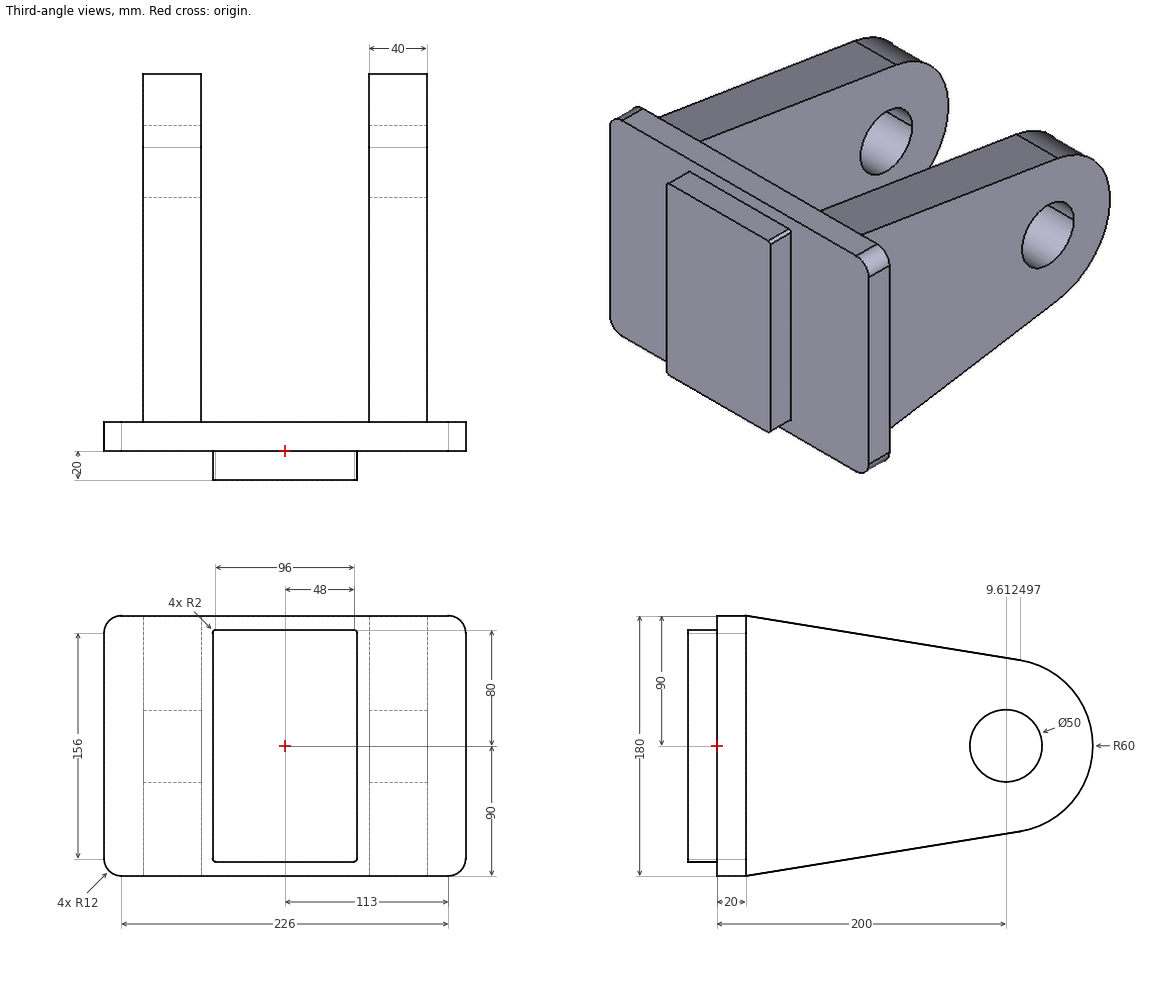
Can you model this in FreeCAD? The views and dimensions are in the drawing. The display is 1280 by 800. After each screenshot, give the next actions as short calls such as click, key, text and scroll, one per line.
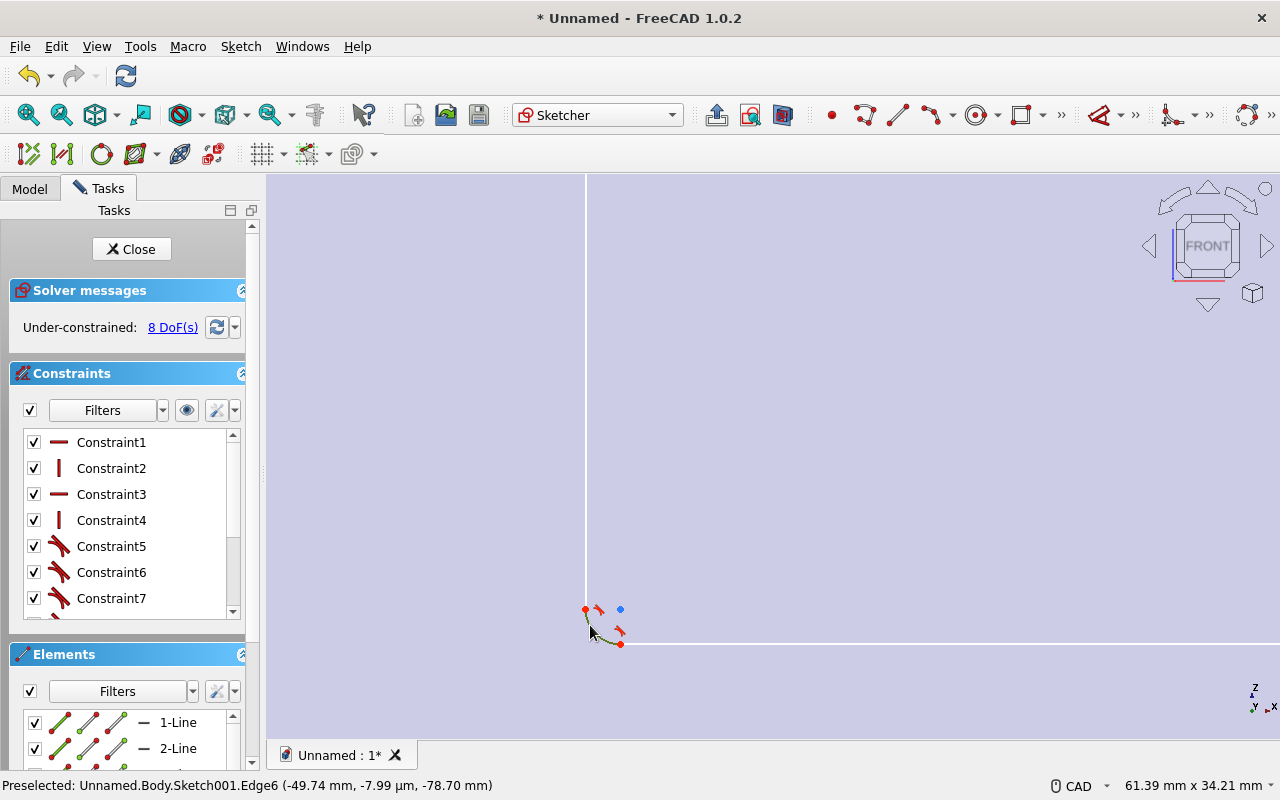
scroll(594, 634, down, 10)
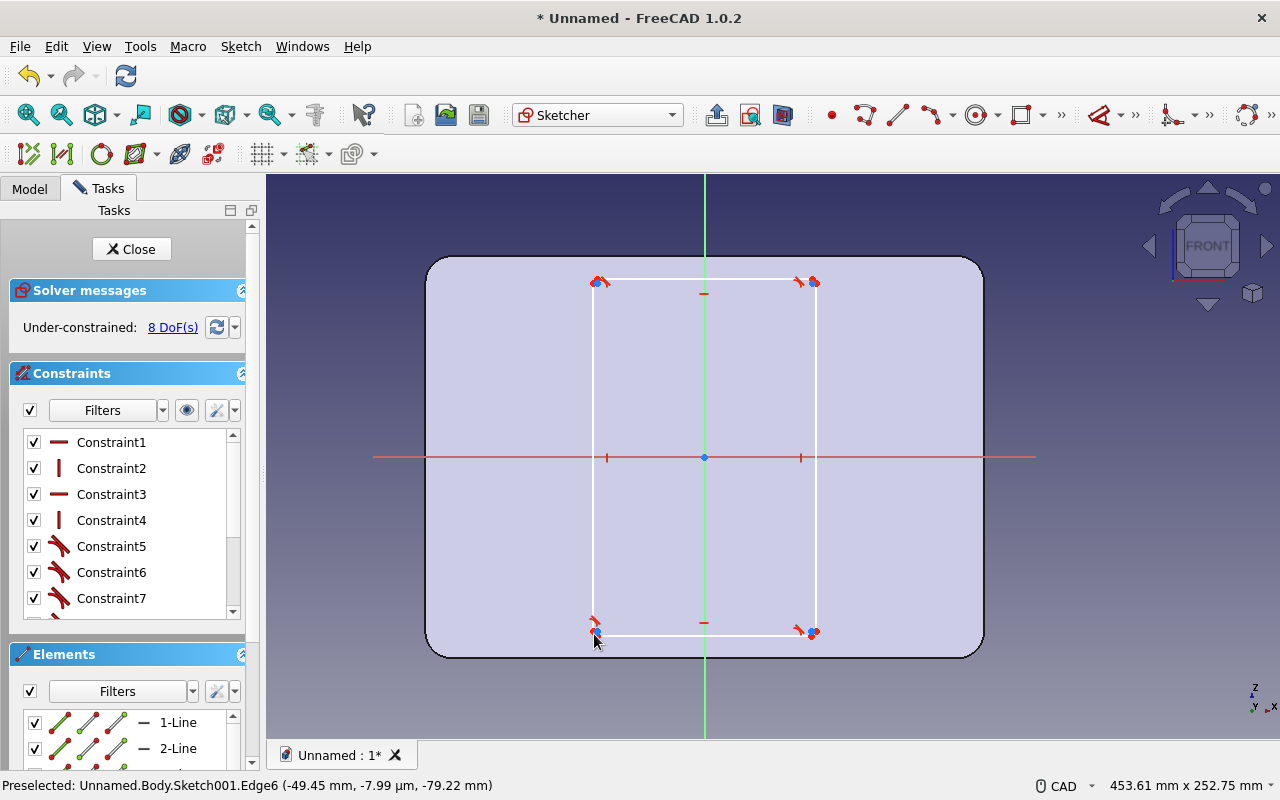
scroll(814, 636, up, 10)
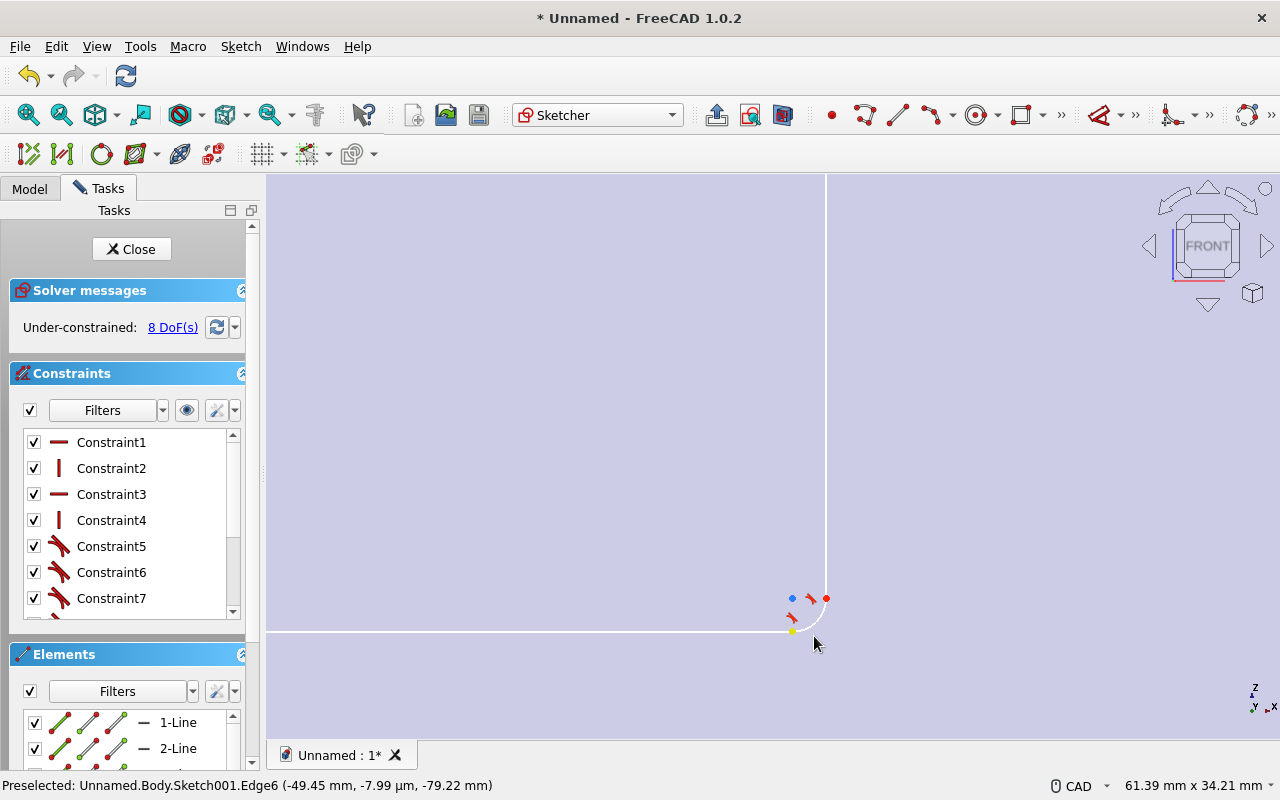
click(808, 628)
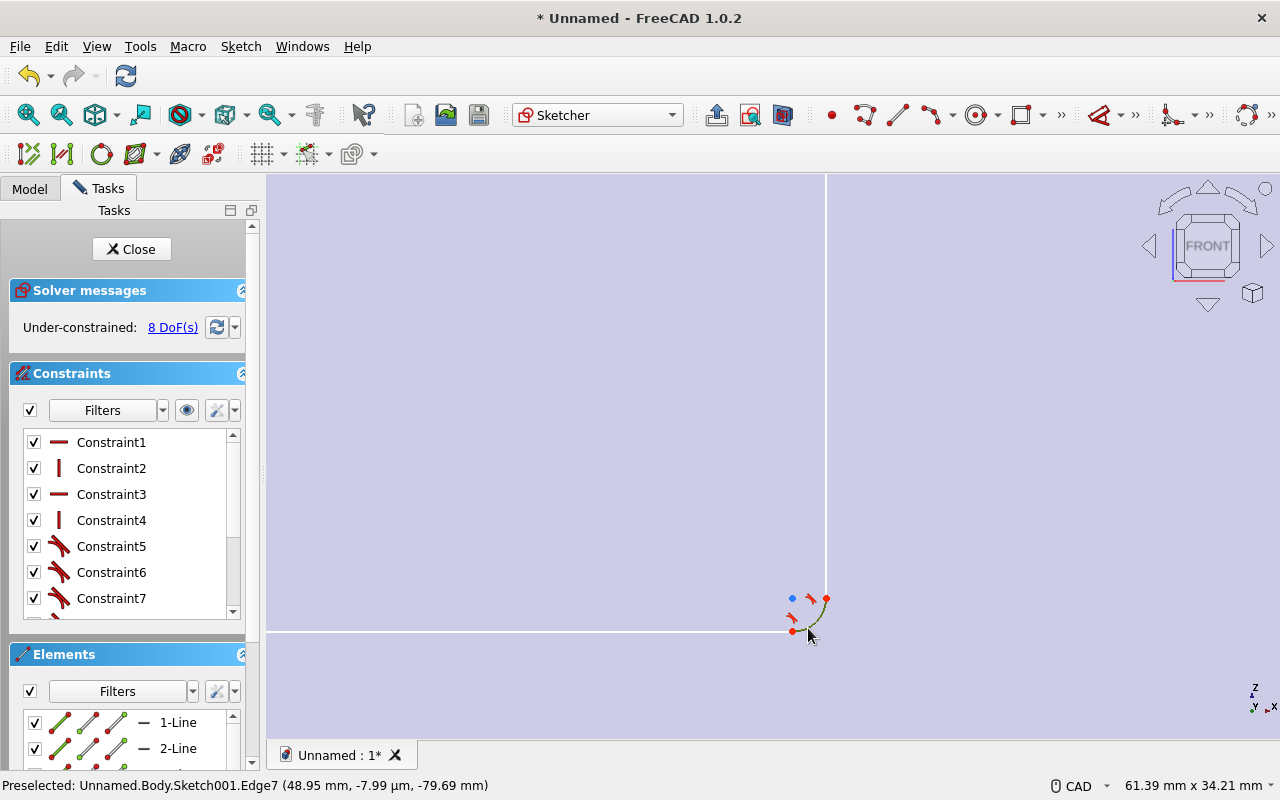
scroll(814, 636, down, 10)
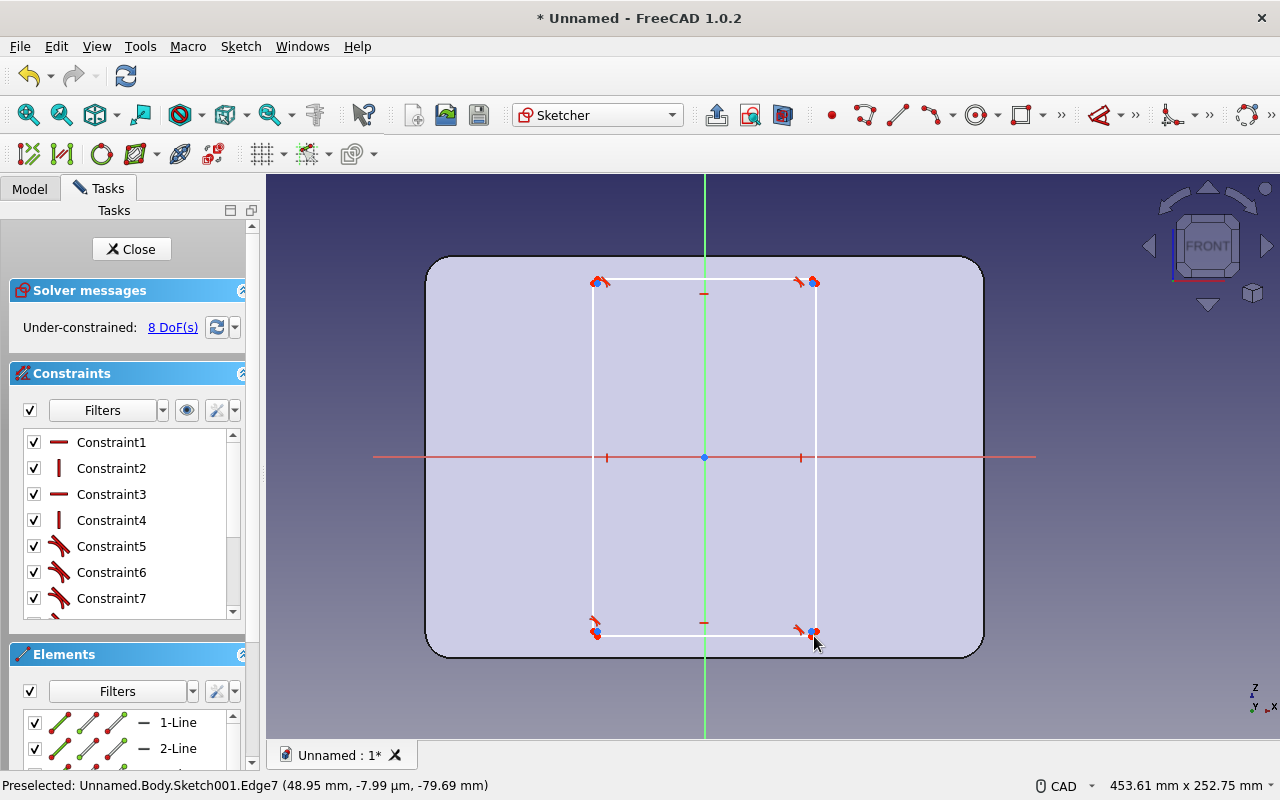
scroll(816, 282, up, 11)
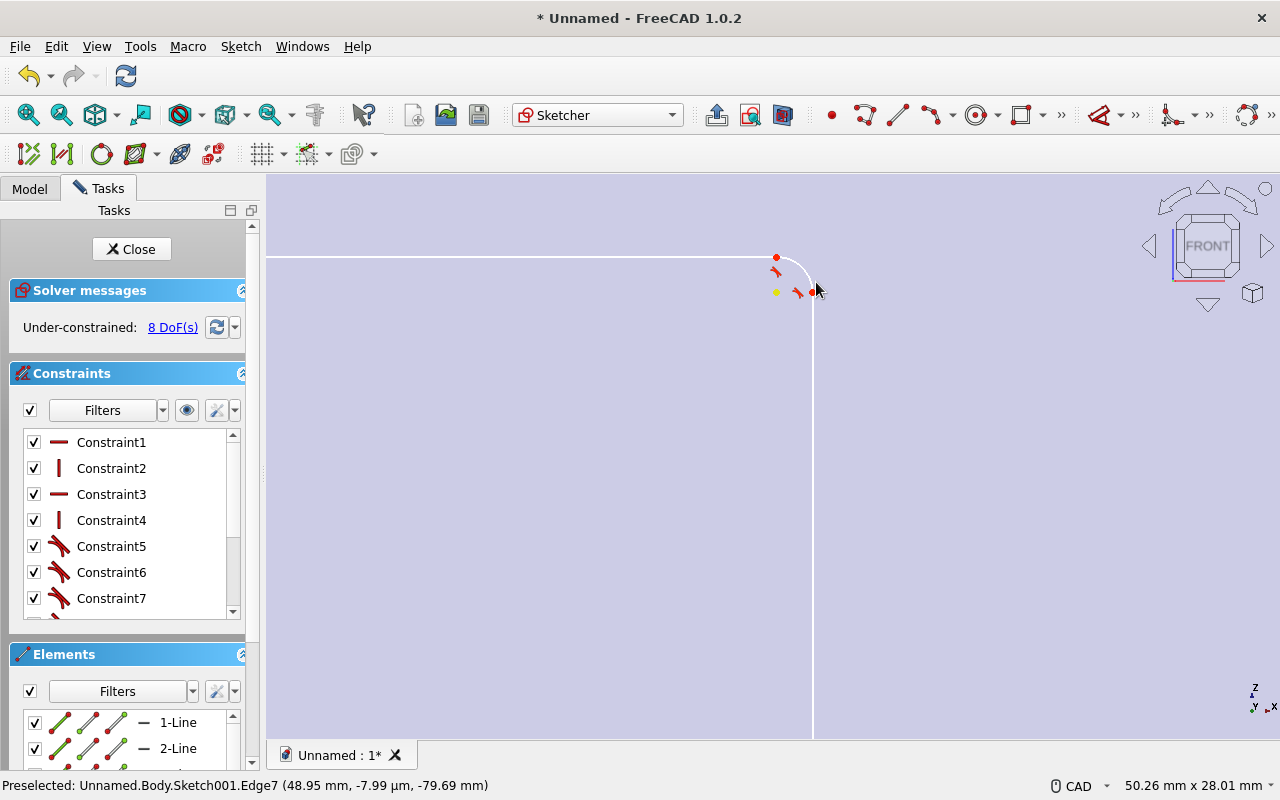
click(809, 277)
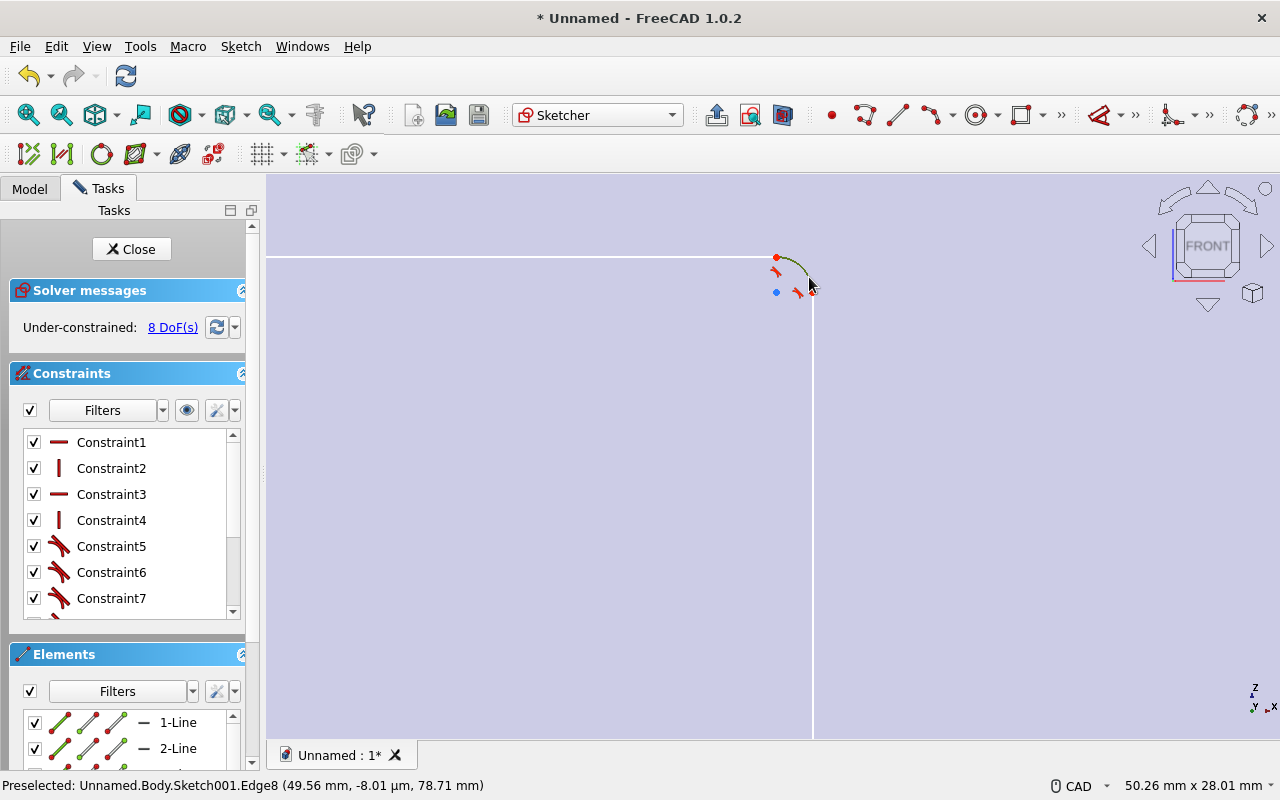
key(e)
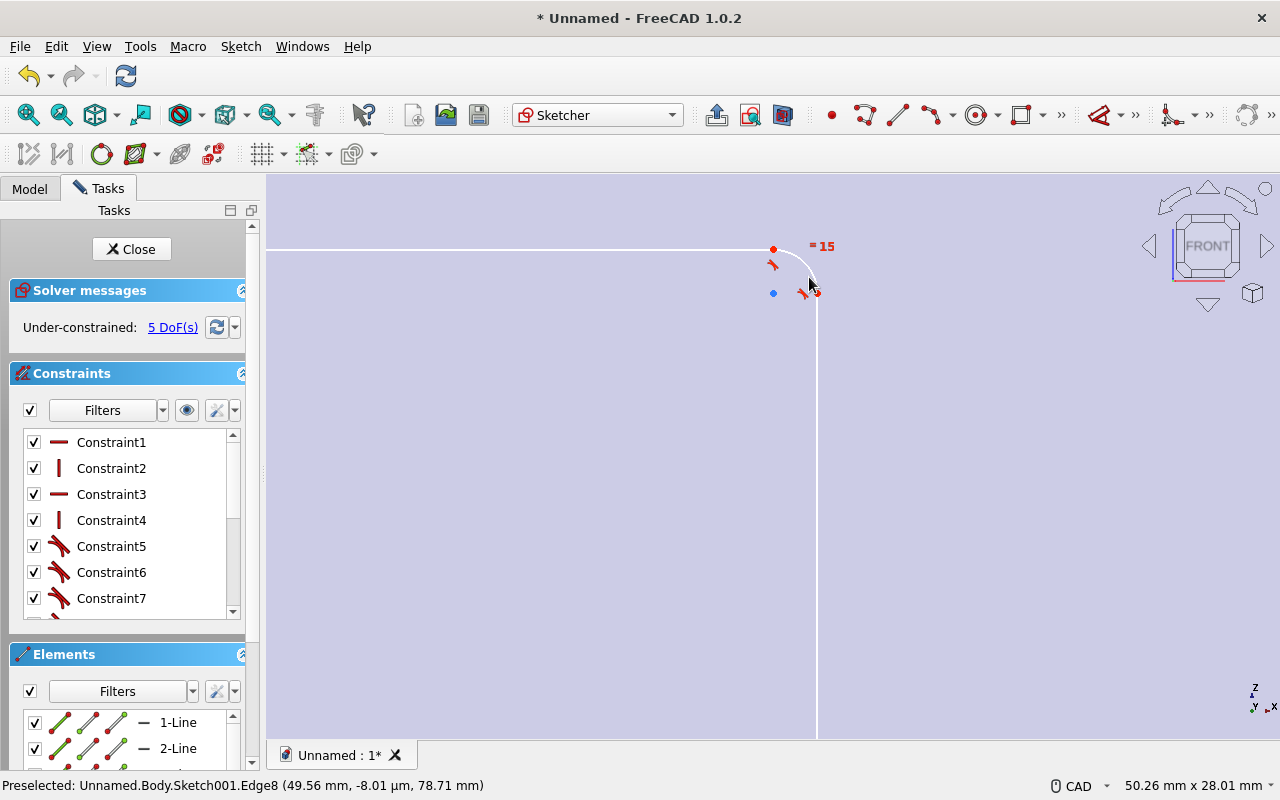
click(1098, 116)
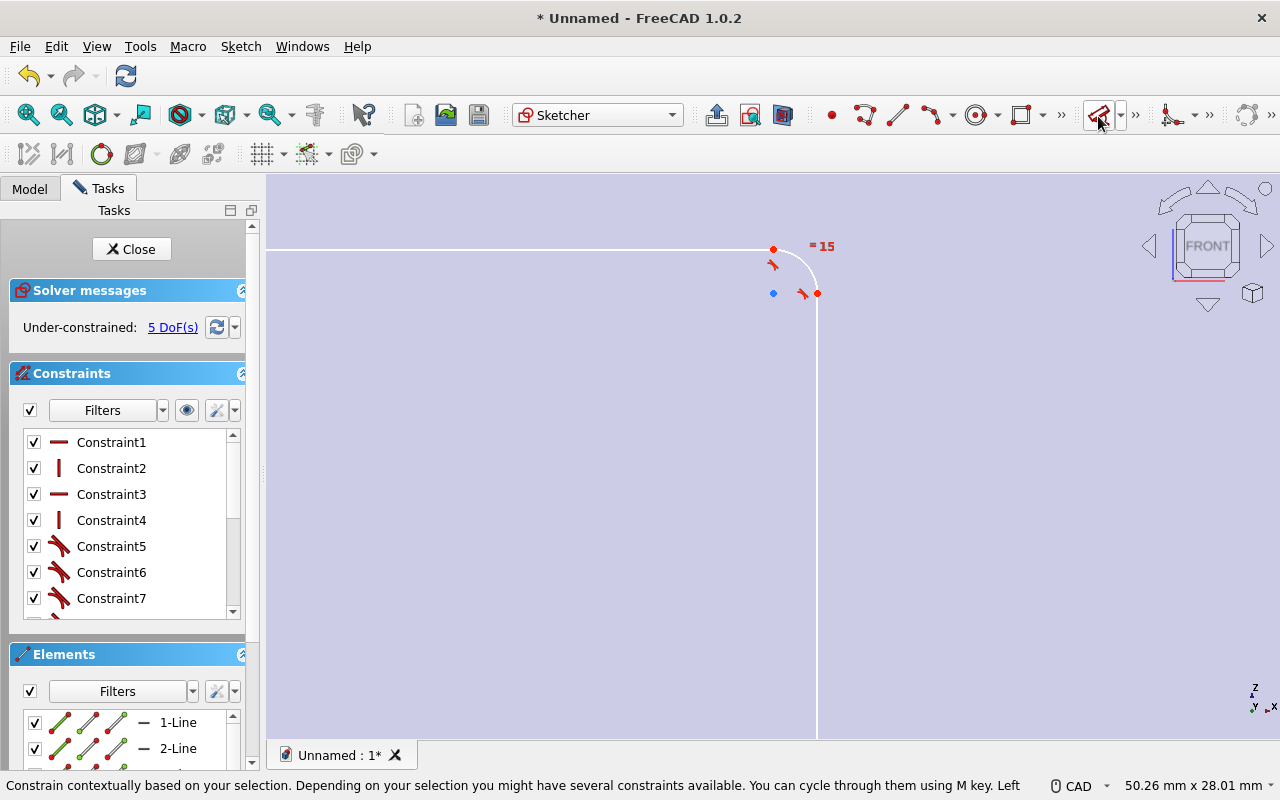
scroll(816, 281, down, 11)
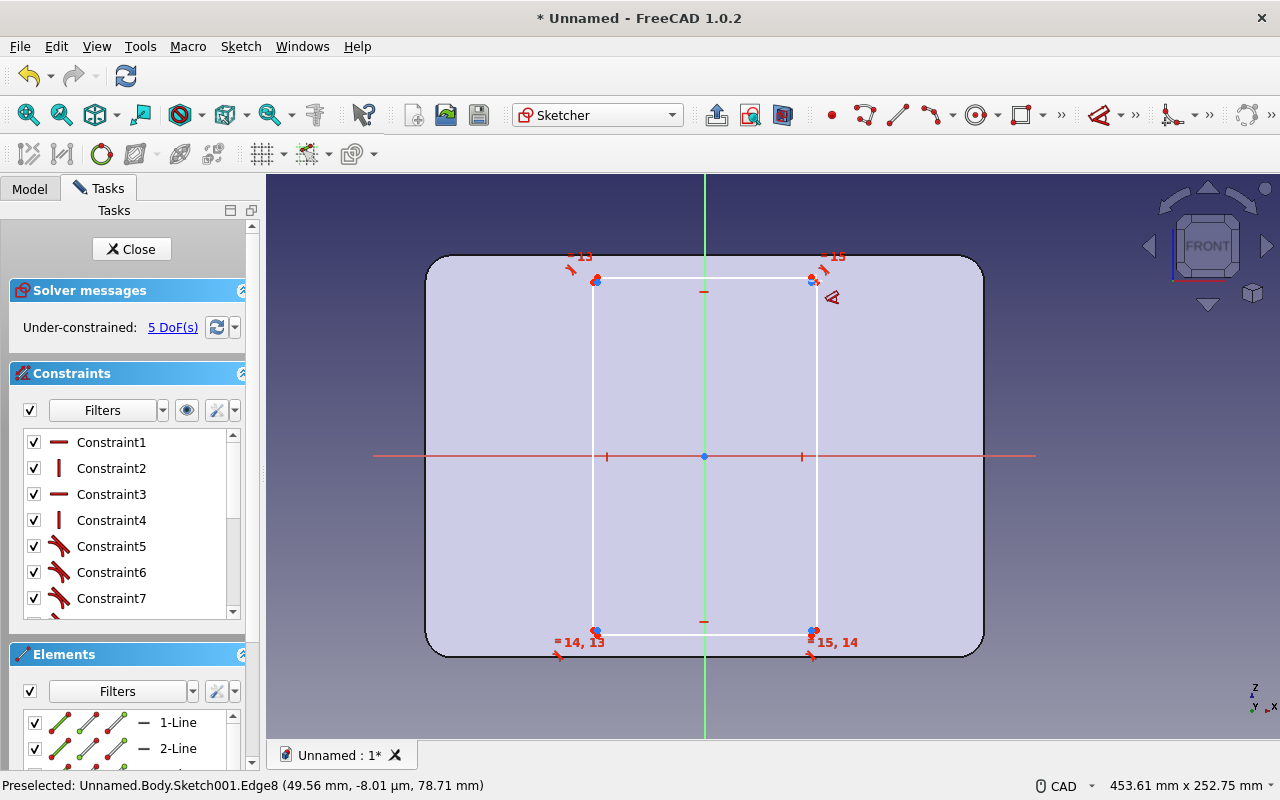
scroll(596, 278, up, 11)